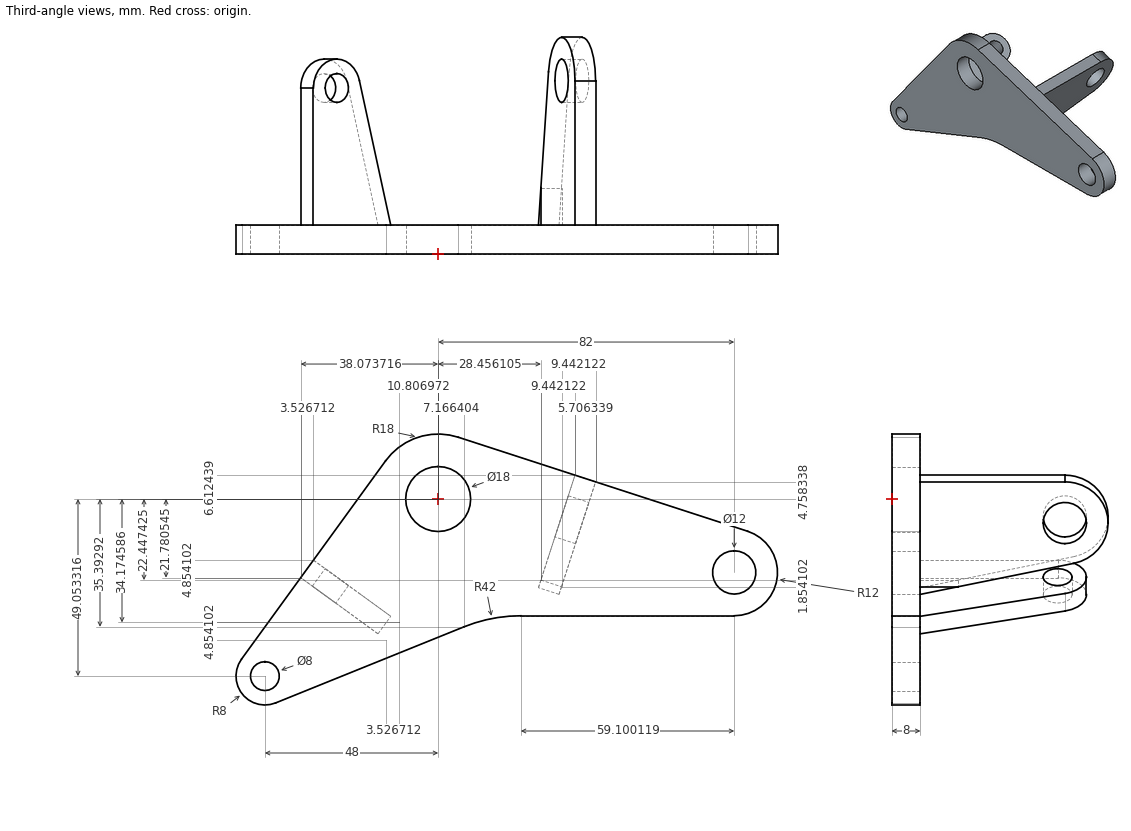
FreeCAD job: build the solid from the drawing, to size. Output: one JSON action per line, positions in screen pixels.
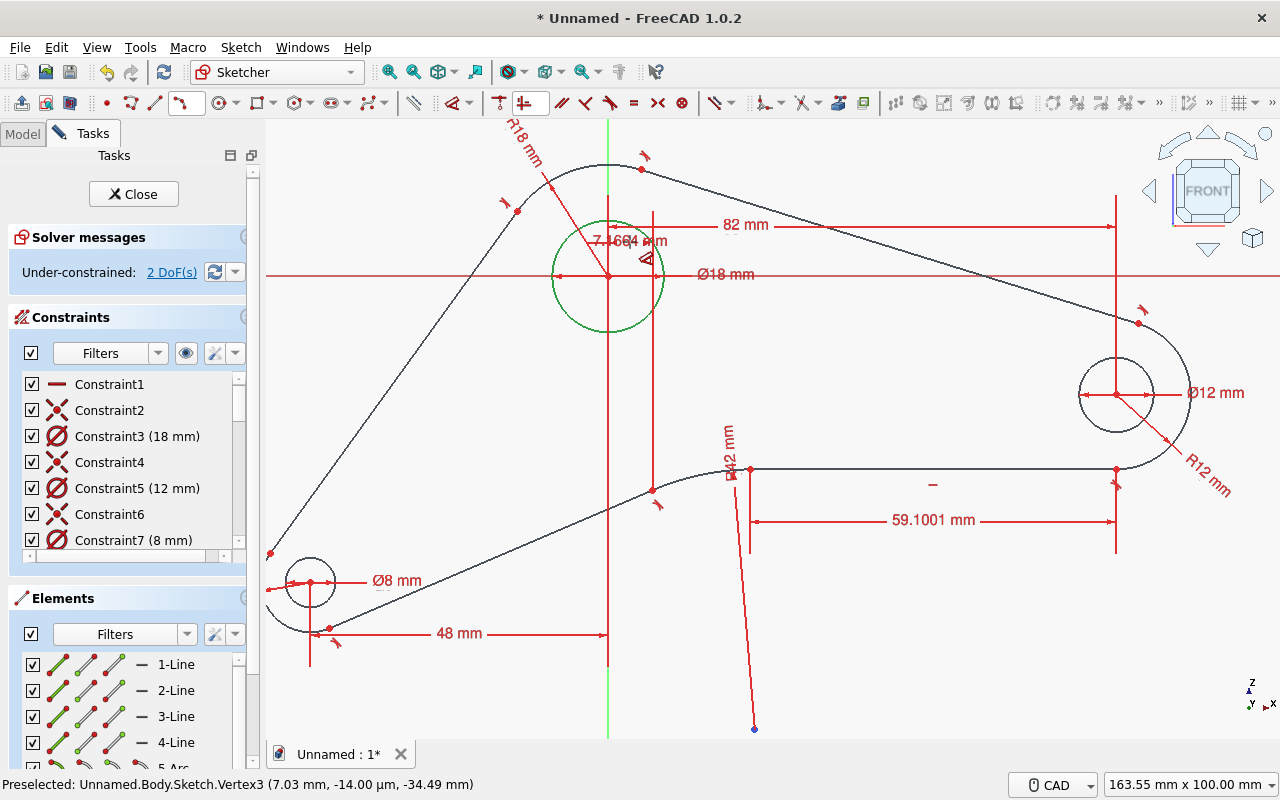
{"action": "left_click", "coordinate": [653, 490]}
{"action": "left_click", "coordinate": [574, 383]}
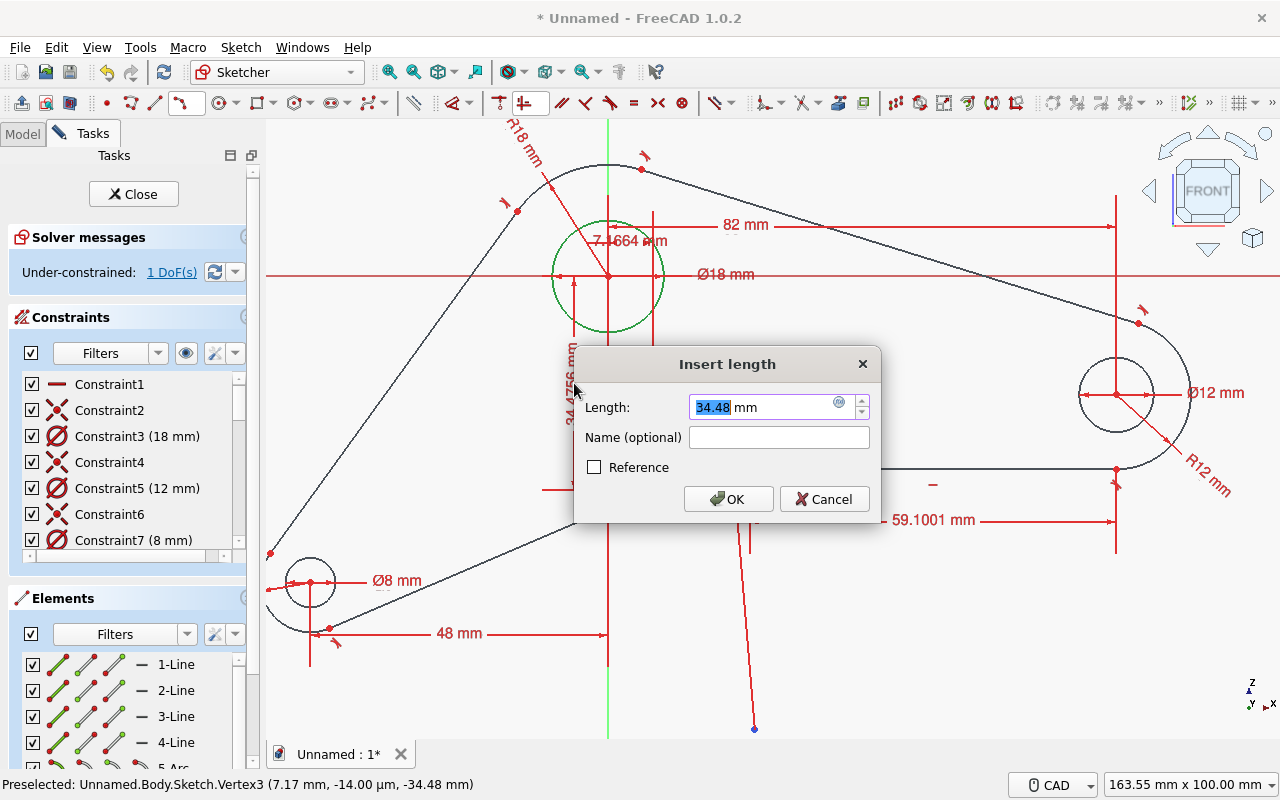
{"action": "type", "text": "35.39292"}
{"action": "key", "text": "Return"}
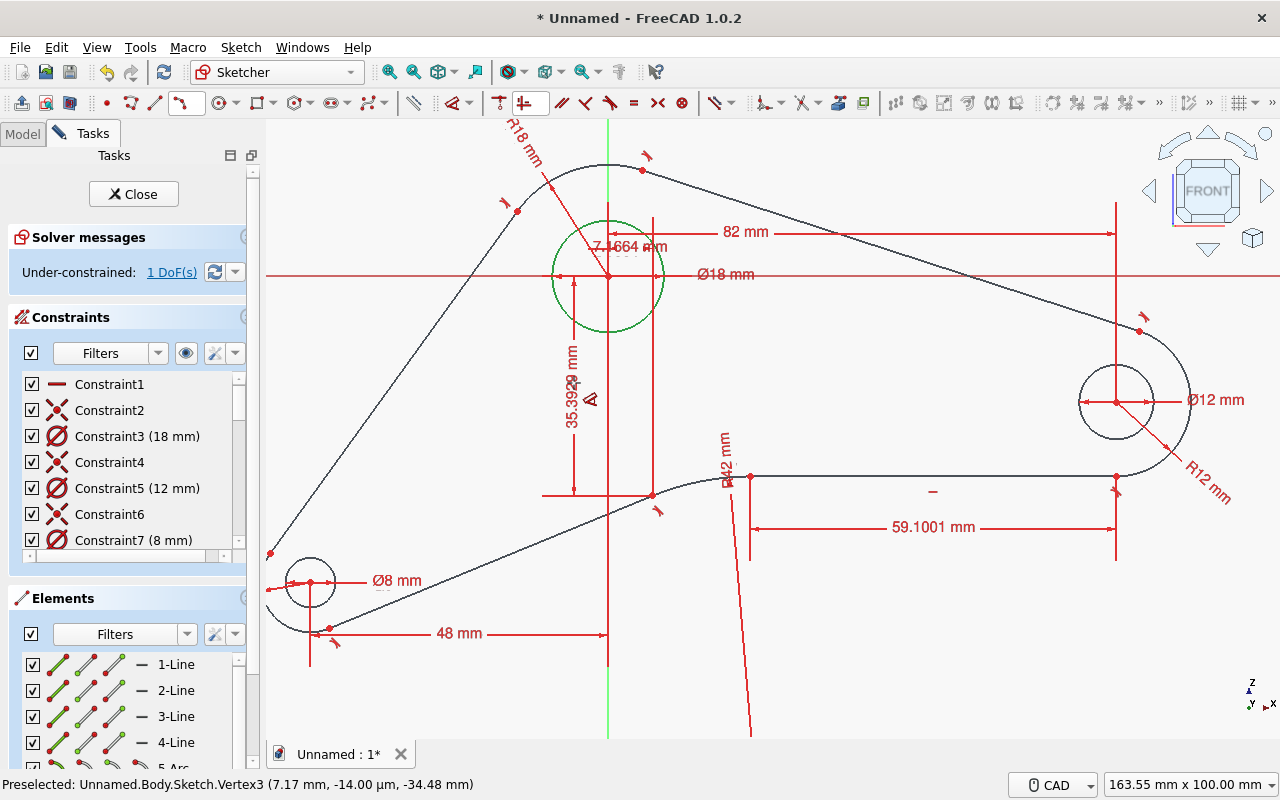
{"action": "left_click", "coordinate": [310, 583]}
{"action": "left_click", "coordinate": [642, 430]}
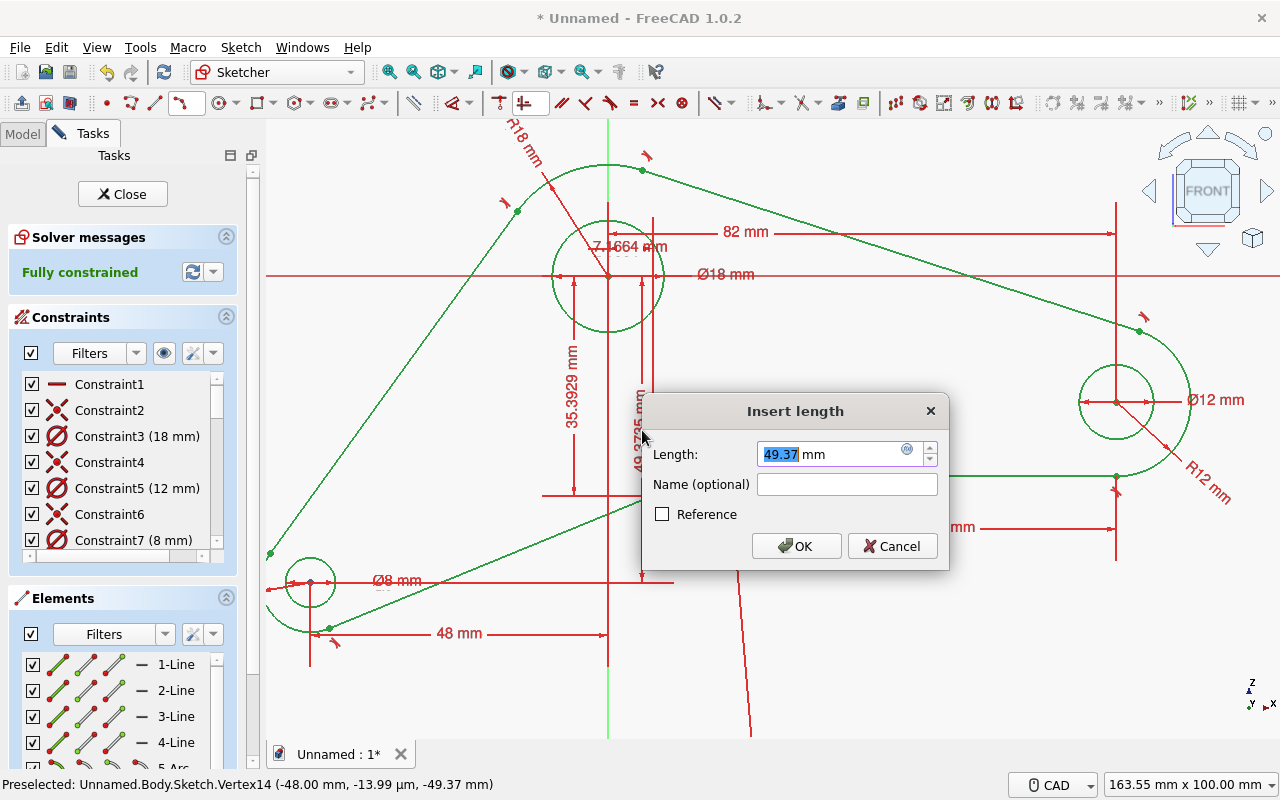
{"action": "type", "text": "49.053316"}
{"action": "key", "text": "Return"}
{"action": "key", "text": "Escape"}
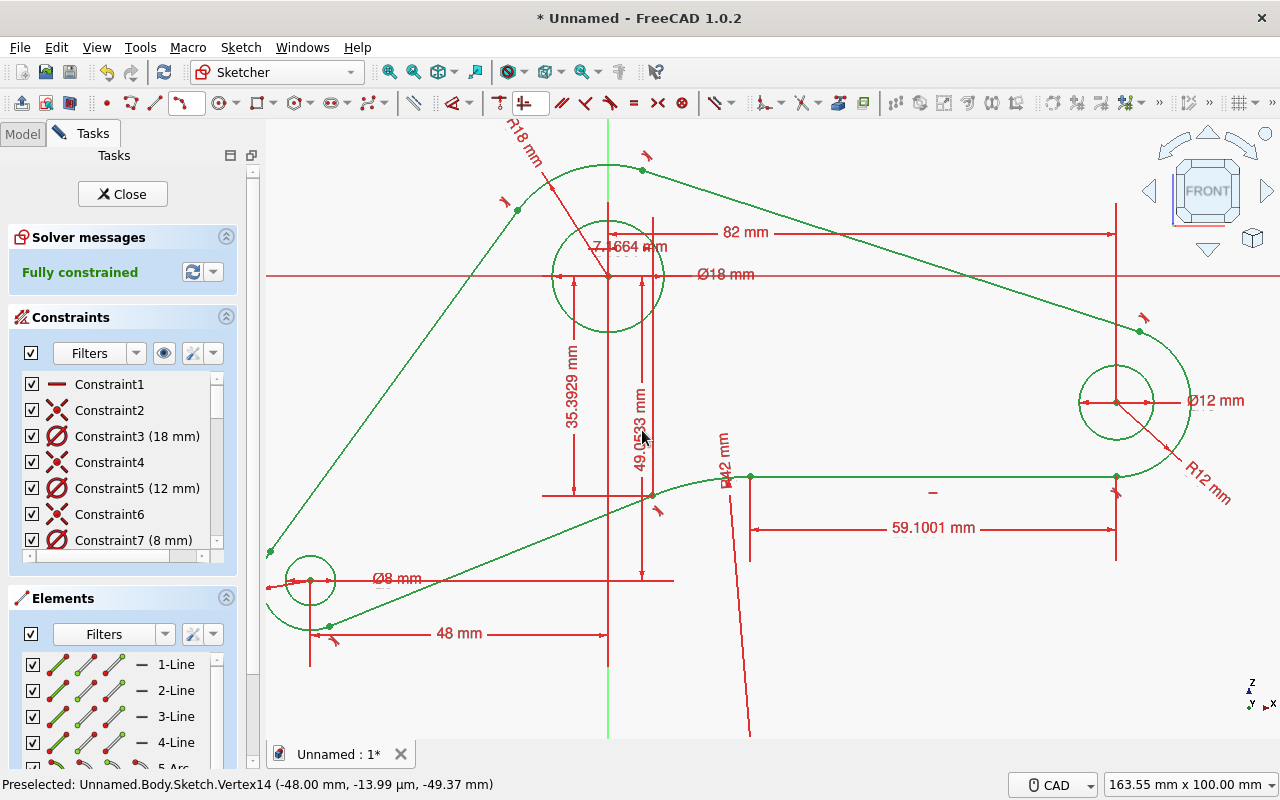
{"action": "left_click", "coordinate": [123, 194]}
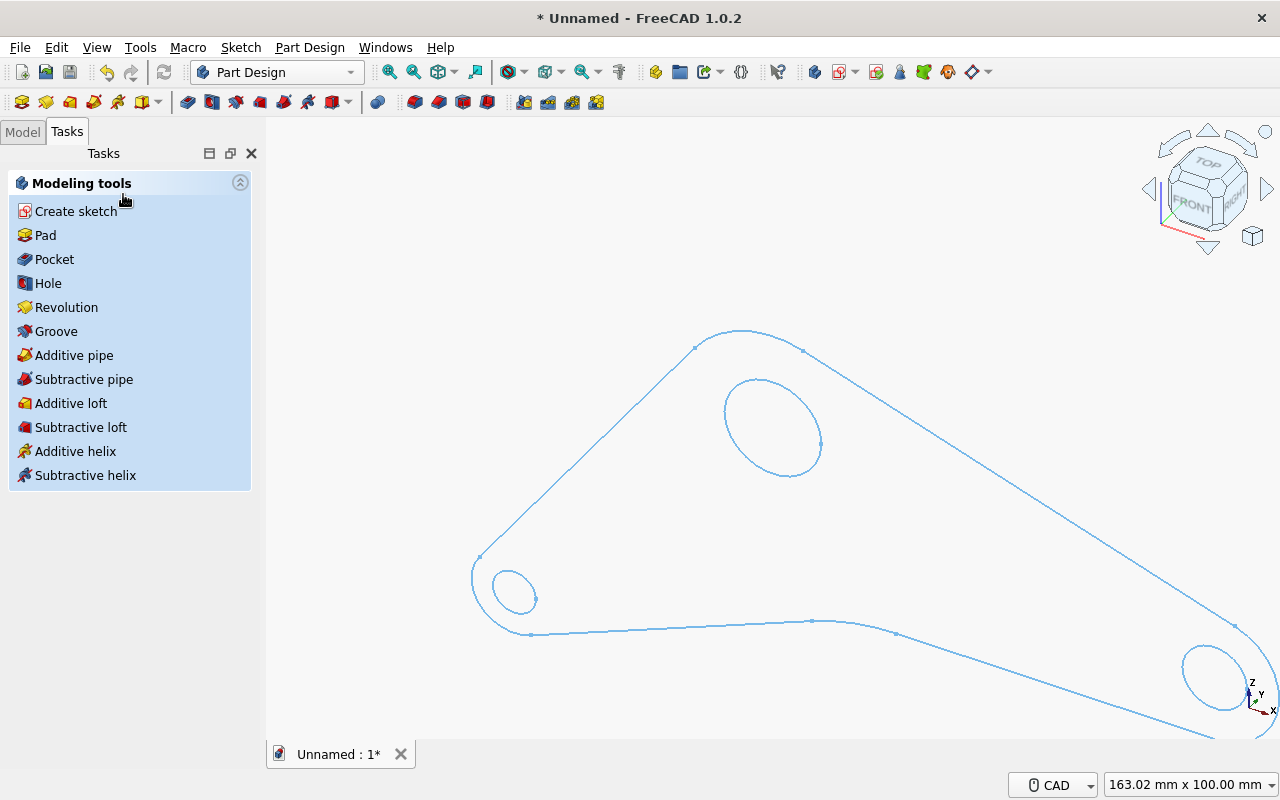
{"action": "left_click", "coordinate": [22, 102]}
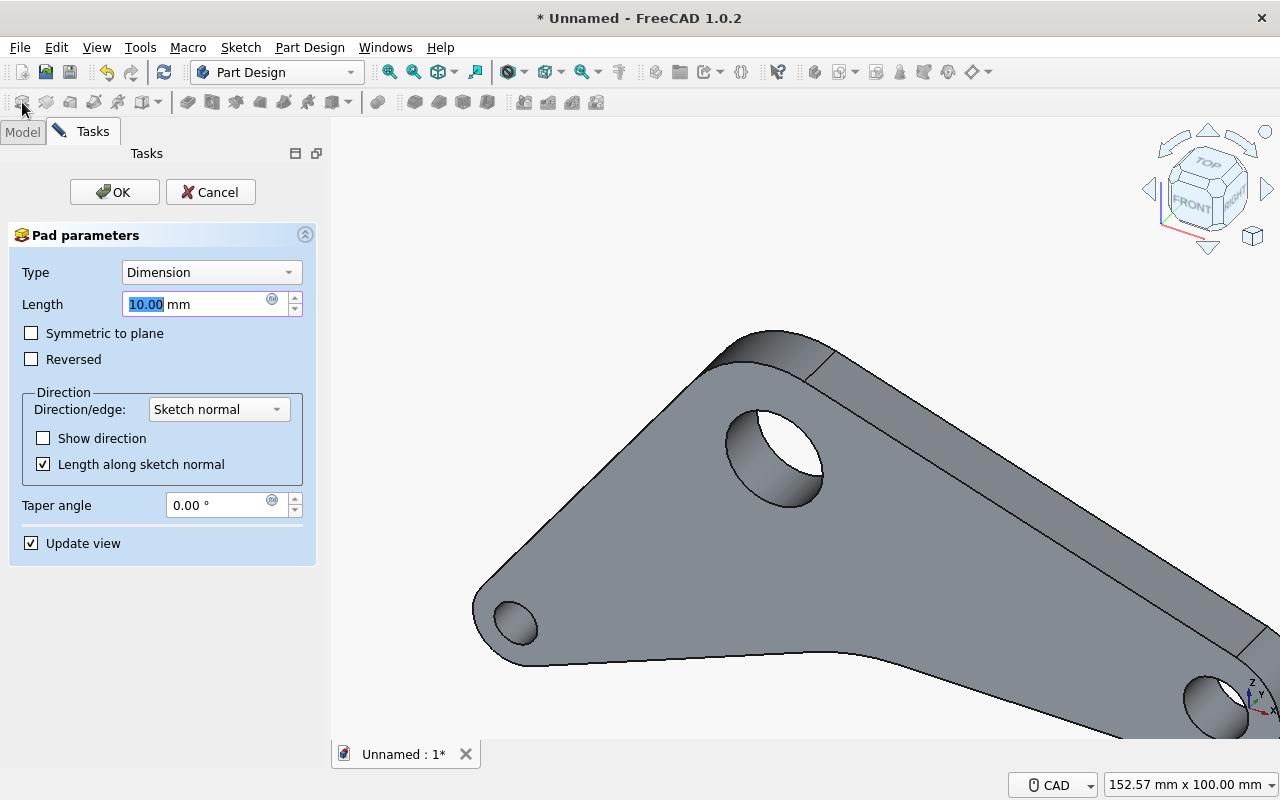
{"action": "type", "text": "8"}
{"action": "key", "text": "Tab"}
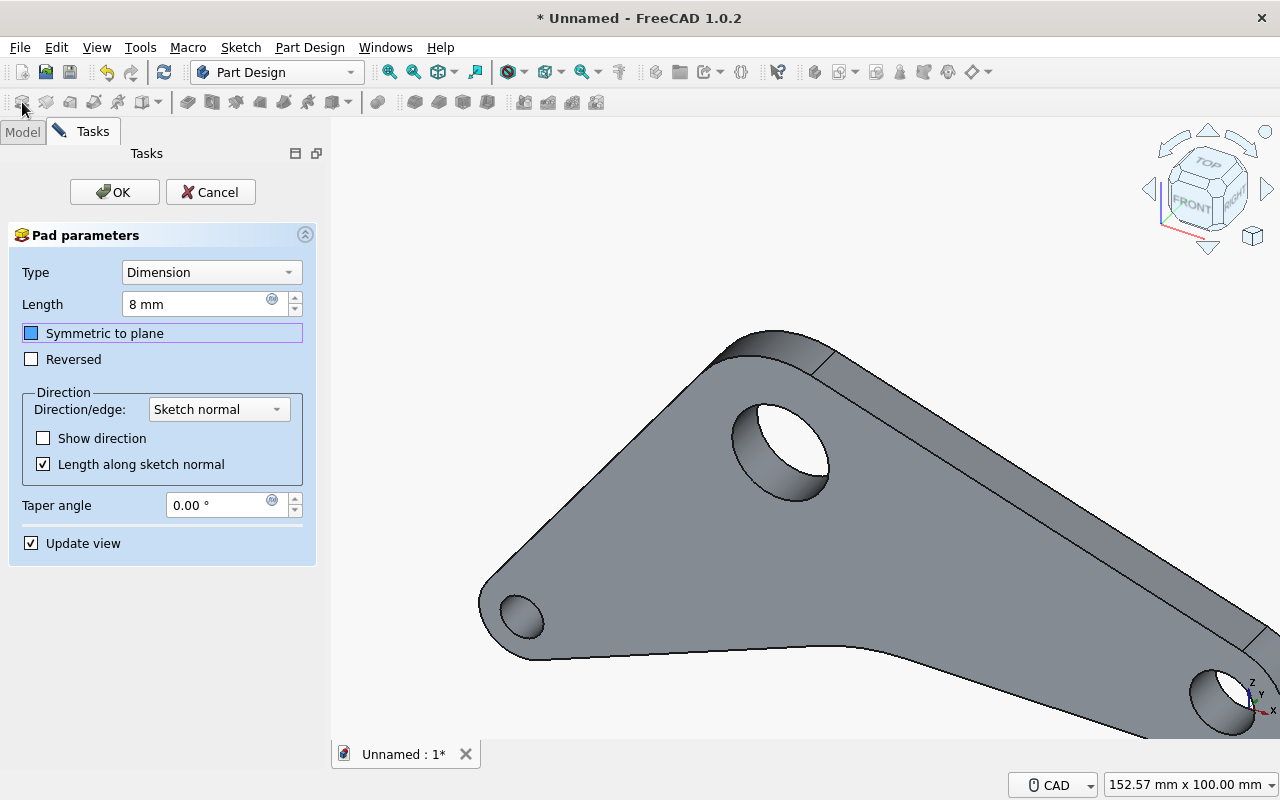
{"action": "left_click", "coordinate": [30, 359]}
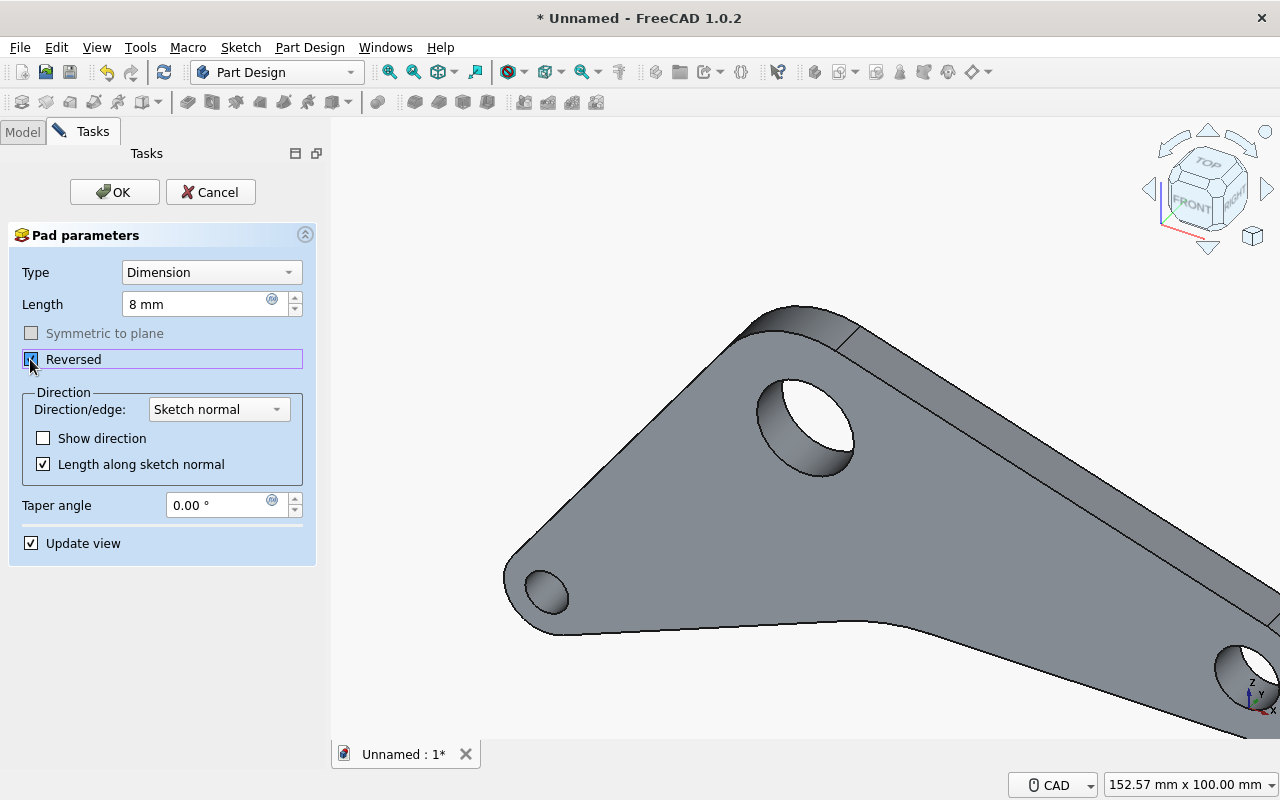
{"action": "left_click", "coordinate": [115, 192]}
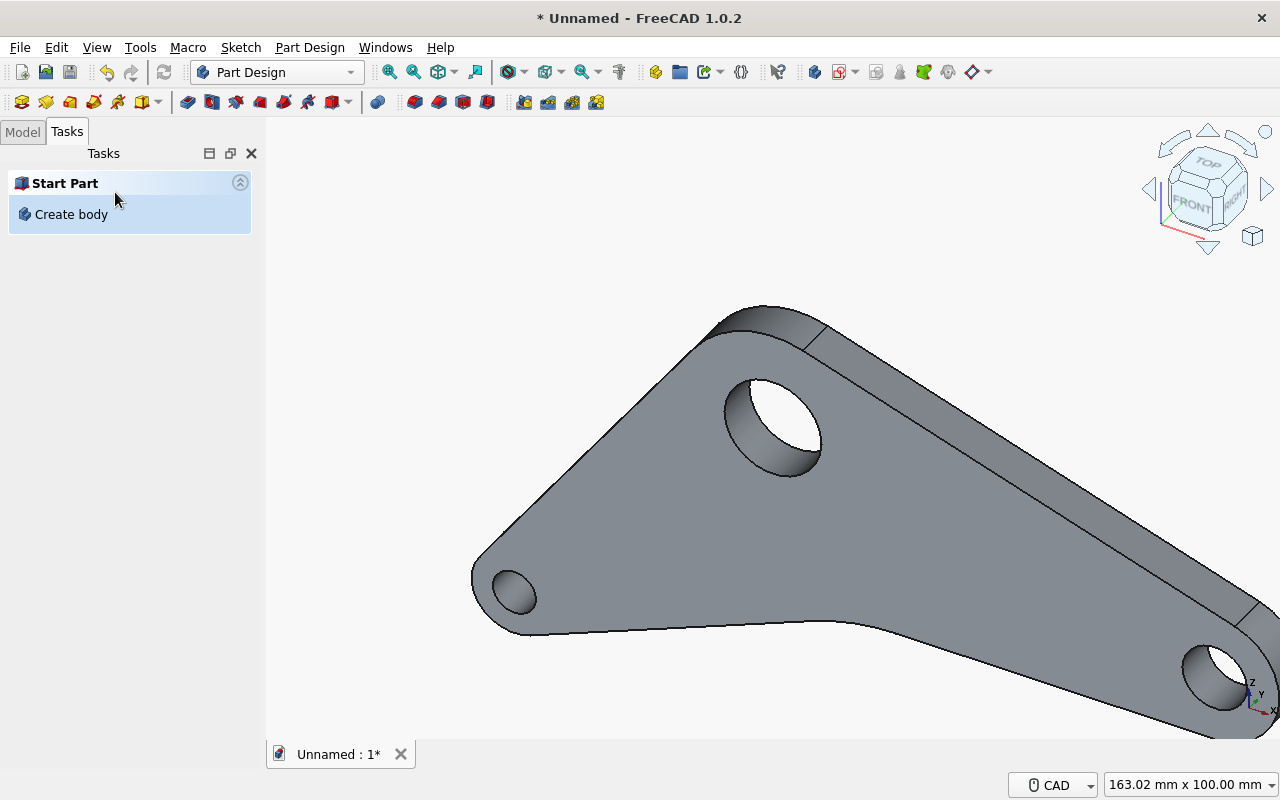
{"action": "left_click", "coordinate": [390, 72]}